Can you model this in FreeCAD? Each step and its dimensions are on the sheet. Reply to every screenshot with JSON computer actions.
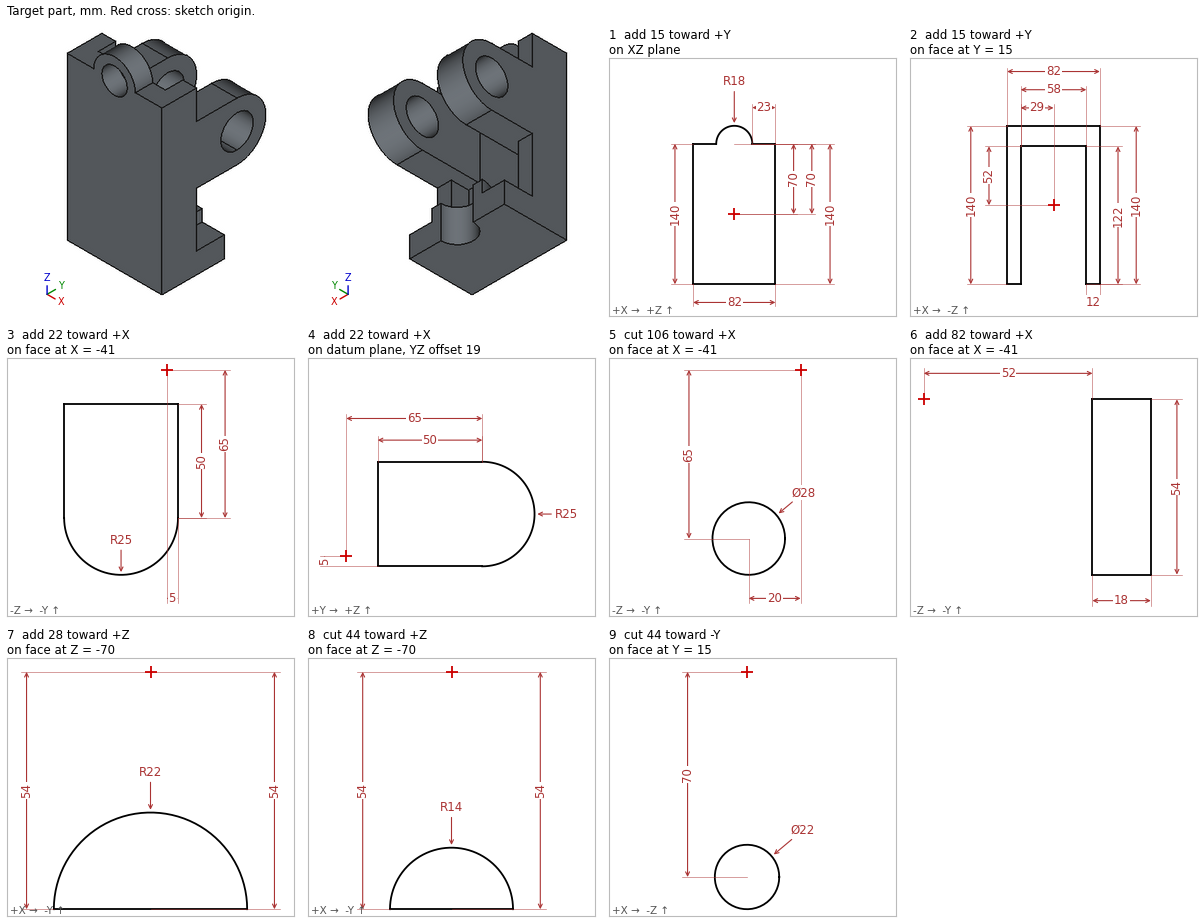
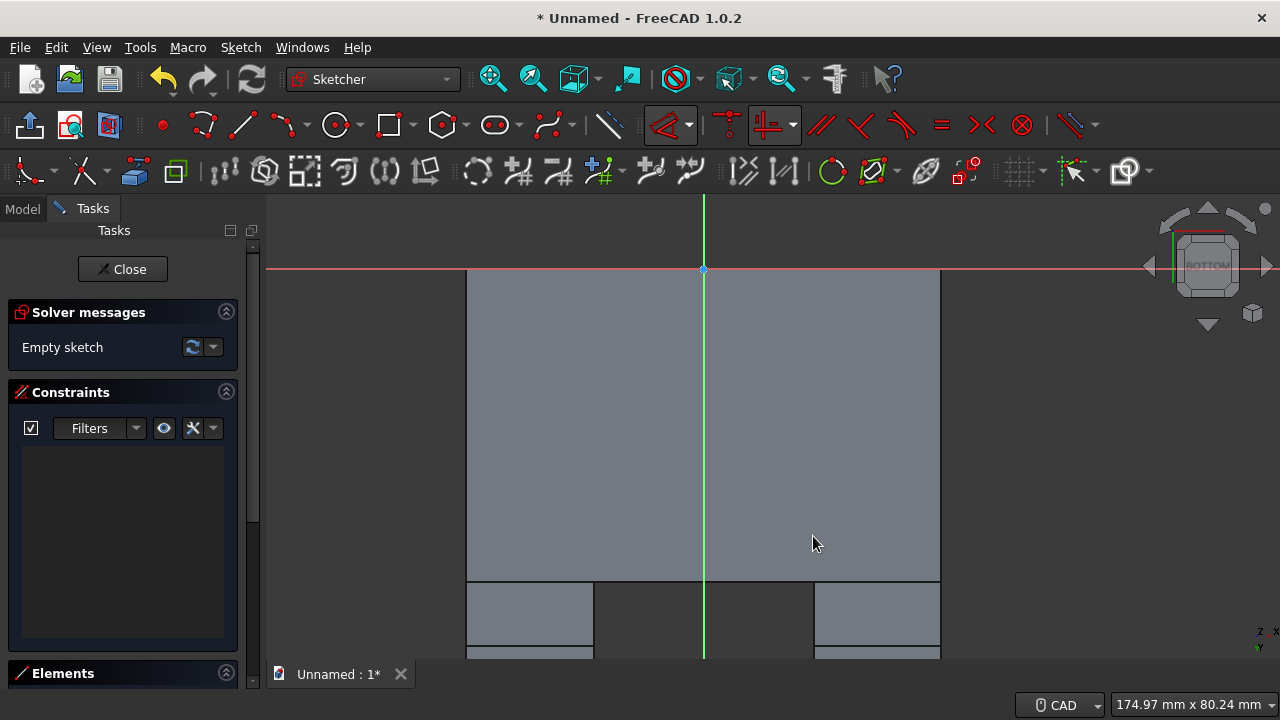
{"action": "key", "text": "g l"}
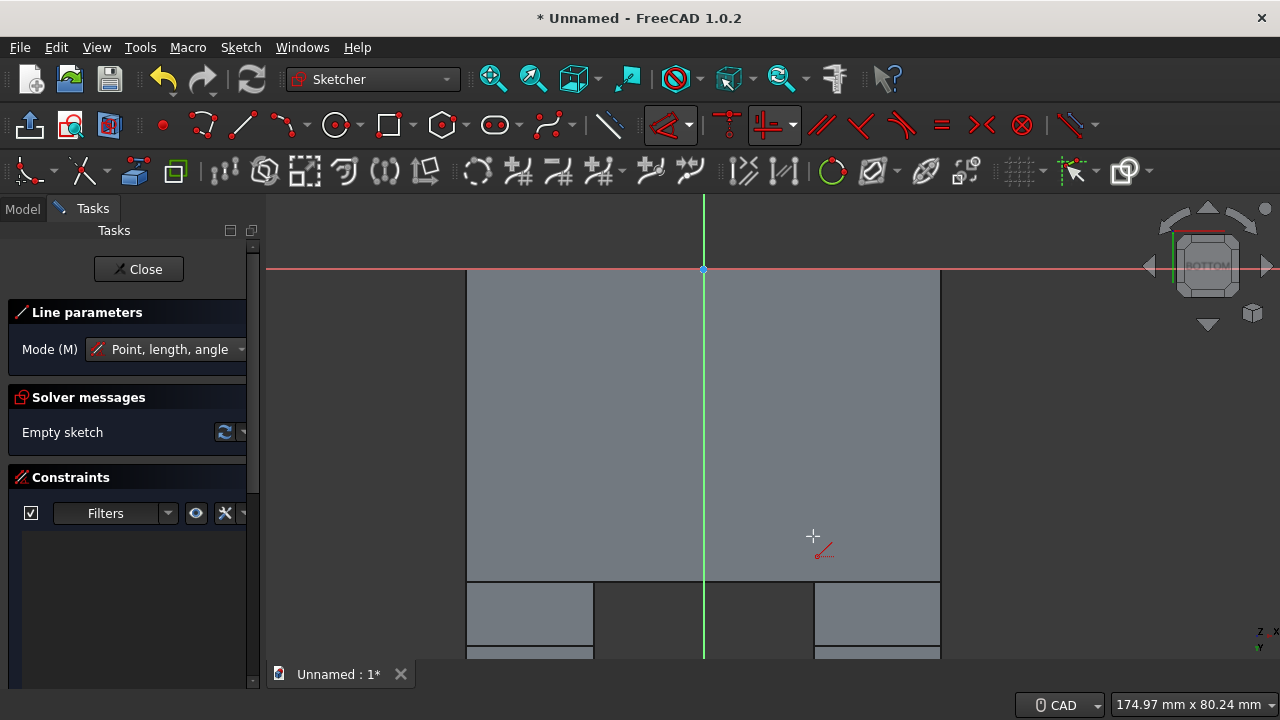
{"action": "left_click", "coordinate": [576, 582]}
{"action": "left_click", "coordinate": [831, 582]}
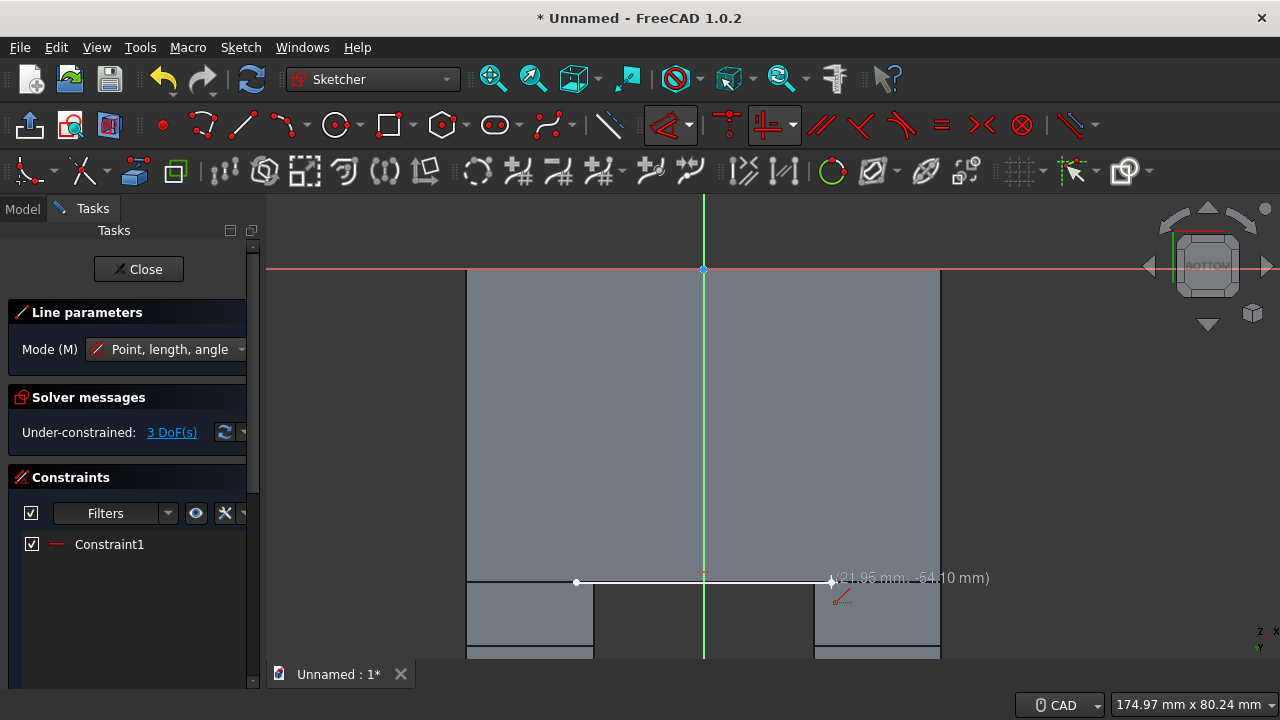
{"action": "left_click", "coordinate": [284, 126]}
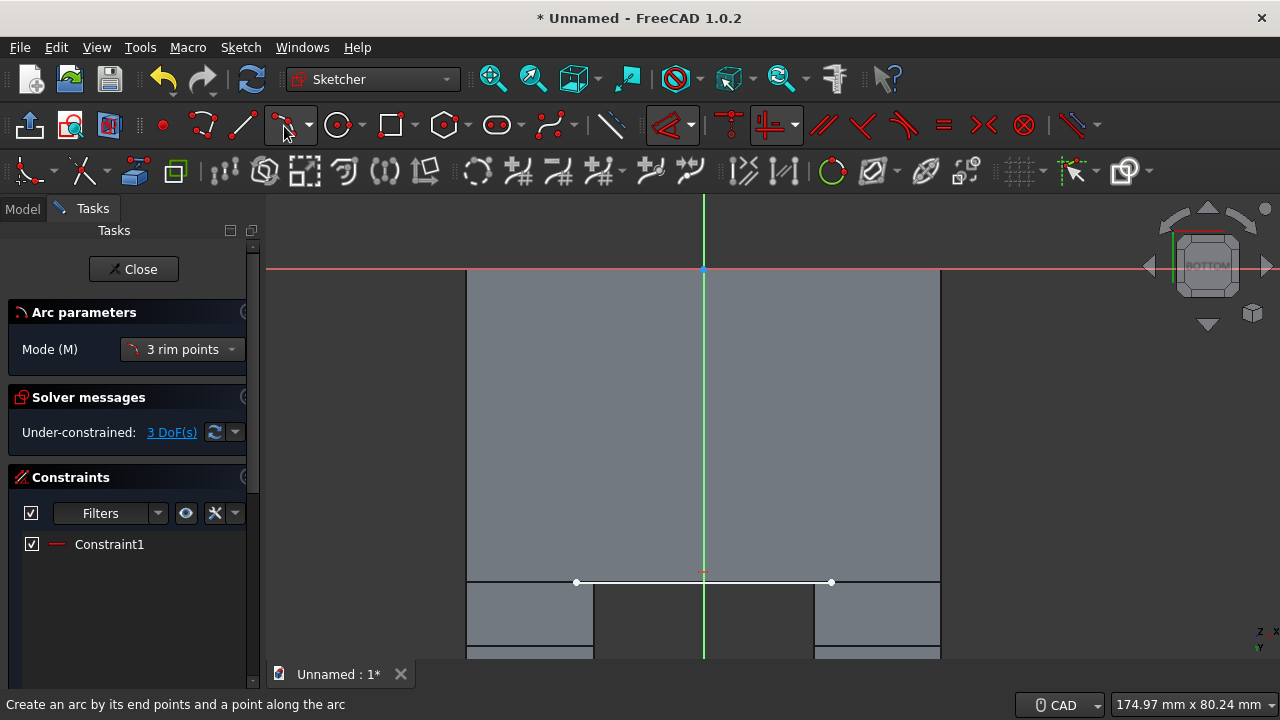
{"action": "left_click", "coordinate": [831, 583]}
{"action": "left_click", "coordinate": [576, 583]}
{"action": "left_click", "coordinate": [743, 461]}
{"action": "key", "text": "Escape"}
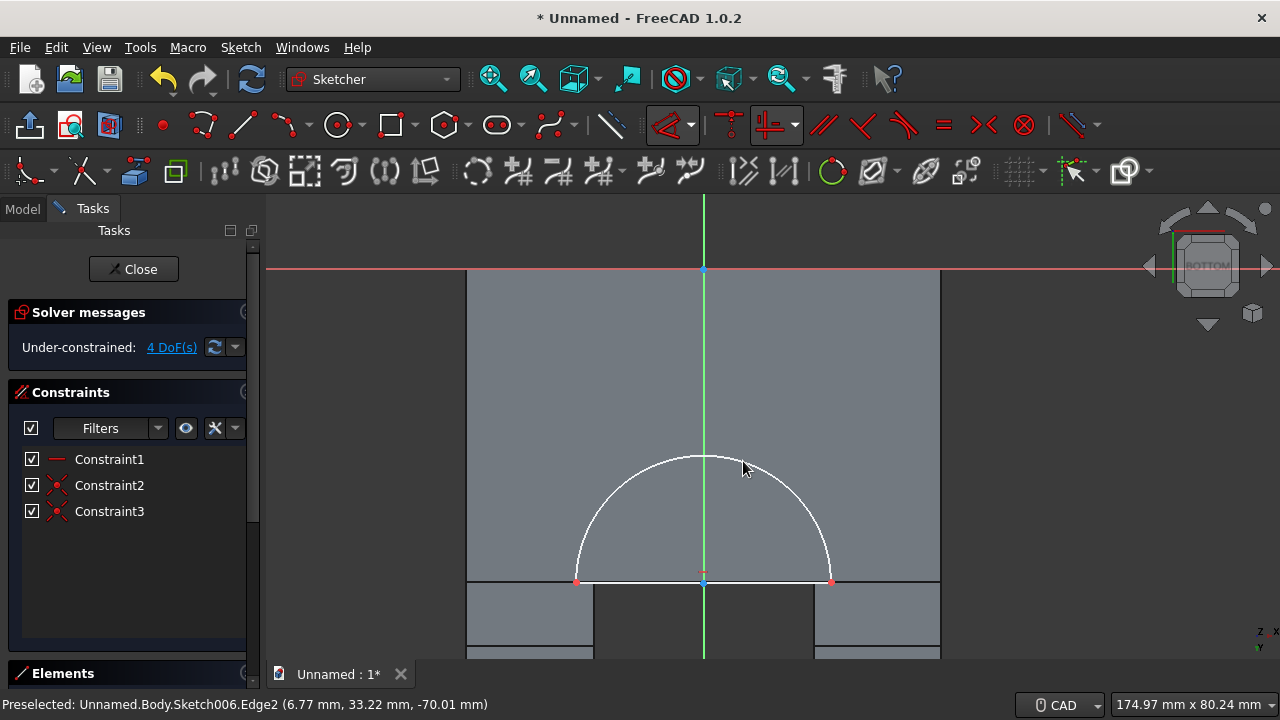
{"action": "left_click", "coordinate": [704, 583]}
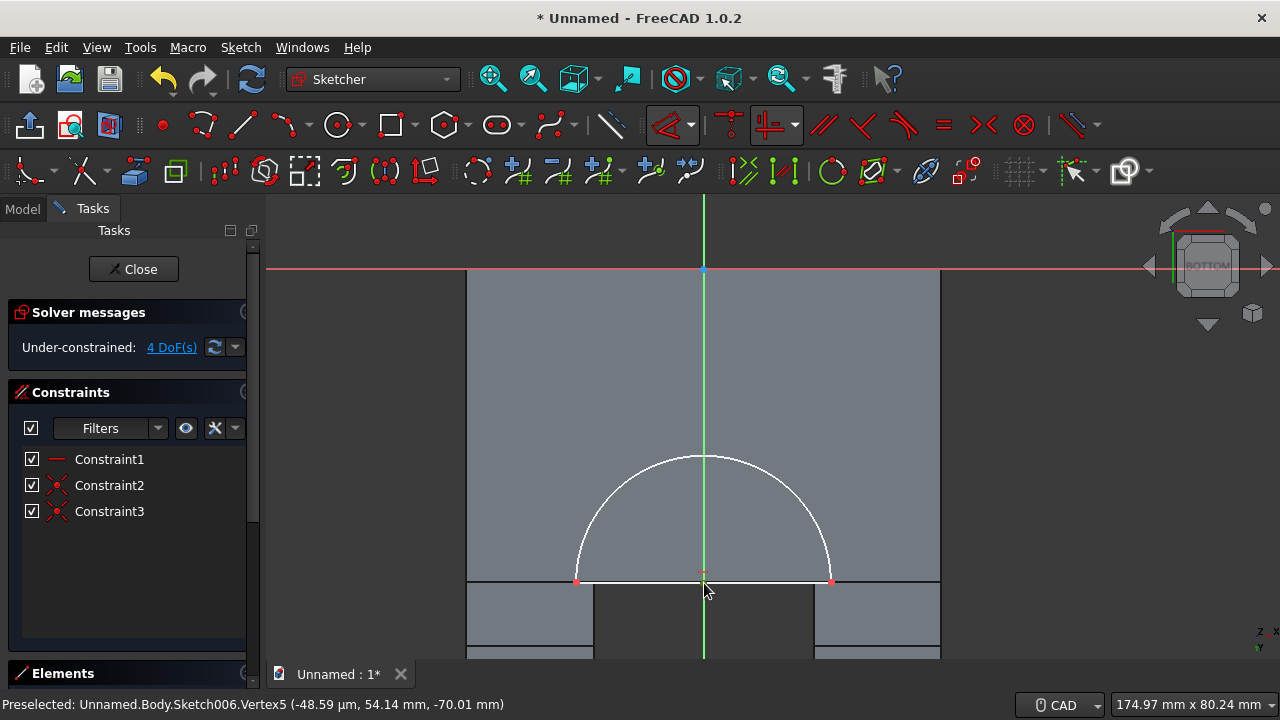
{"action": "left_click", "coordinate": [704, 543]}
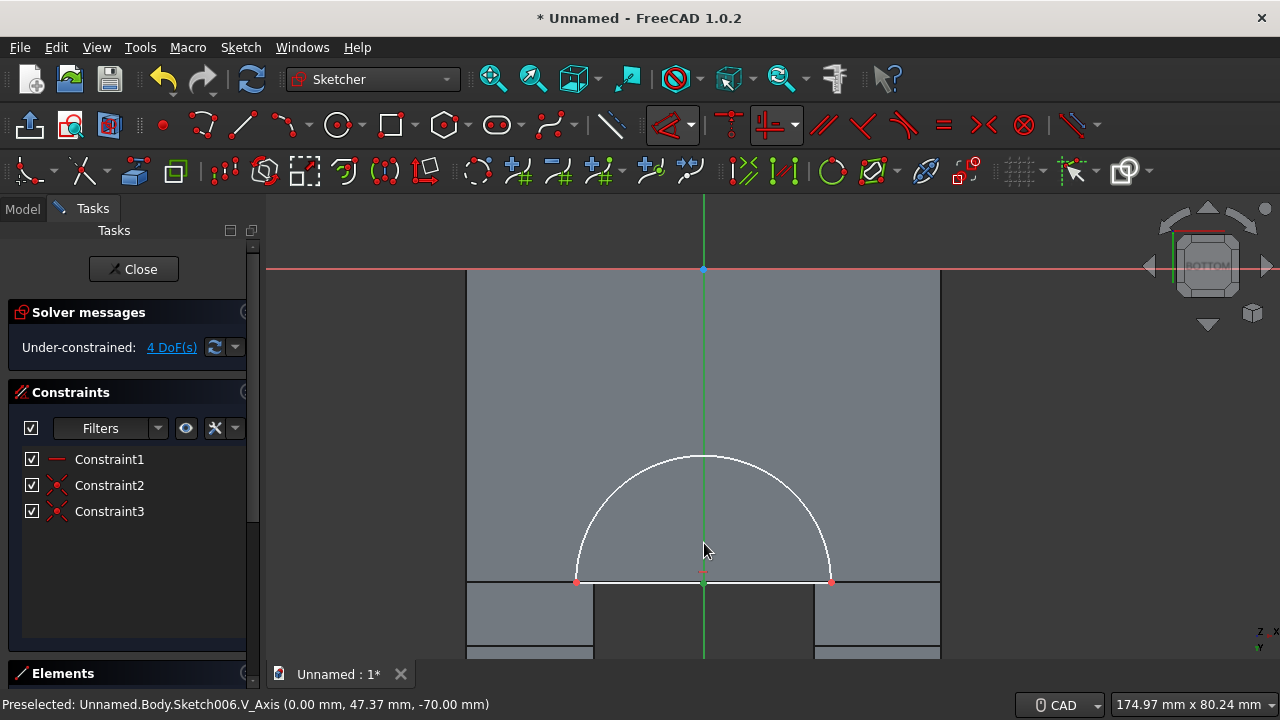
{"action": "left_click", "coordinate": [730, 126]}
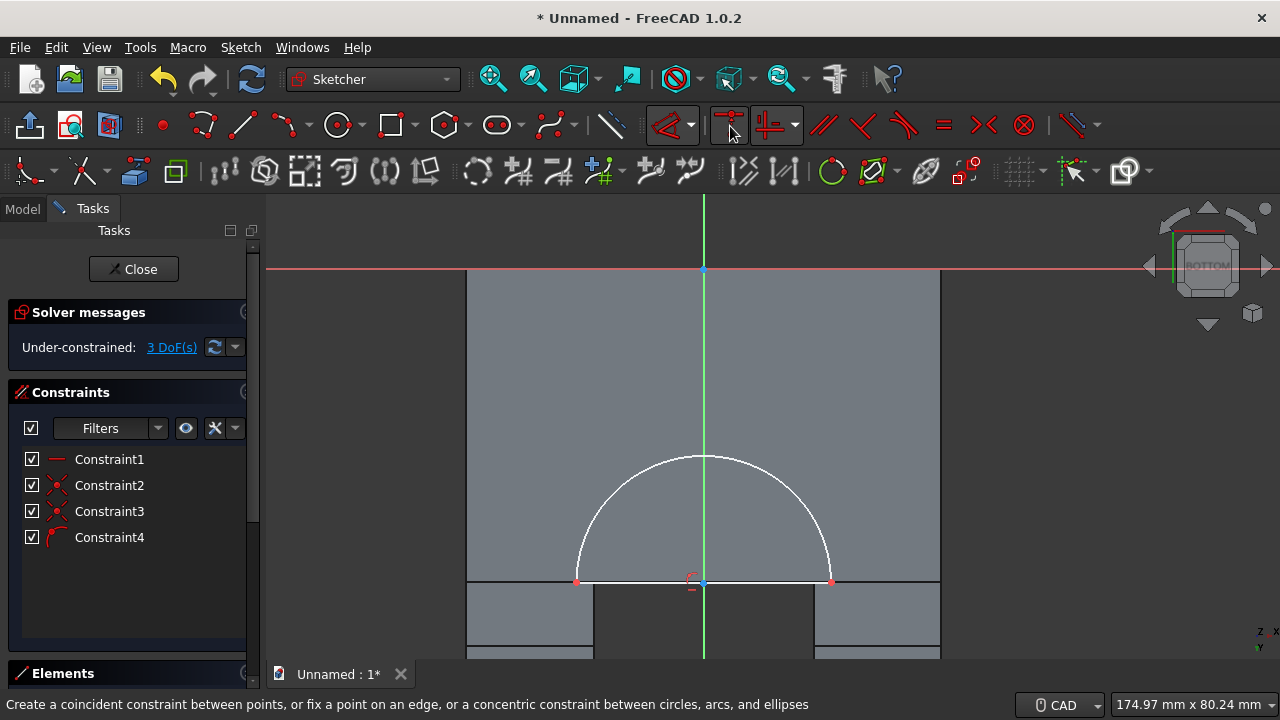
{"action": "left_click", "coordinate": [779, 480]}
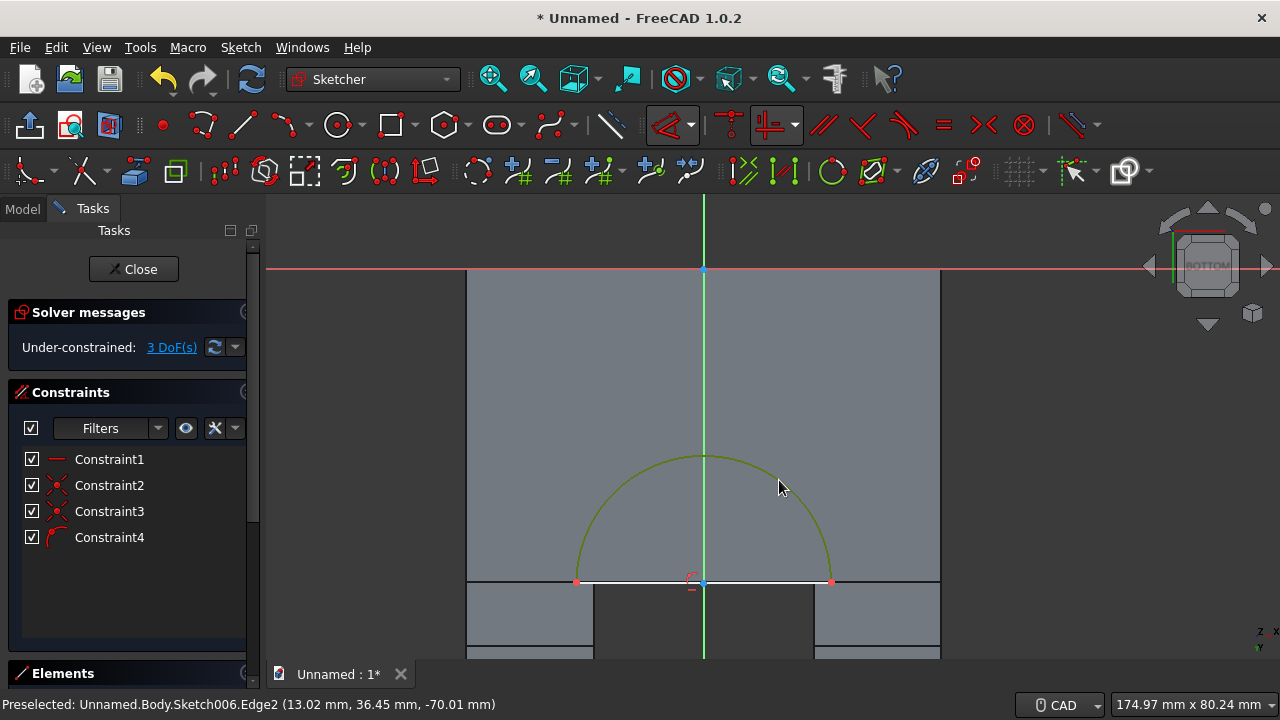
{"action": "key", "text": "k r"}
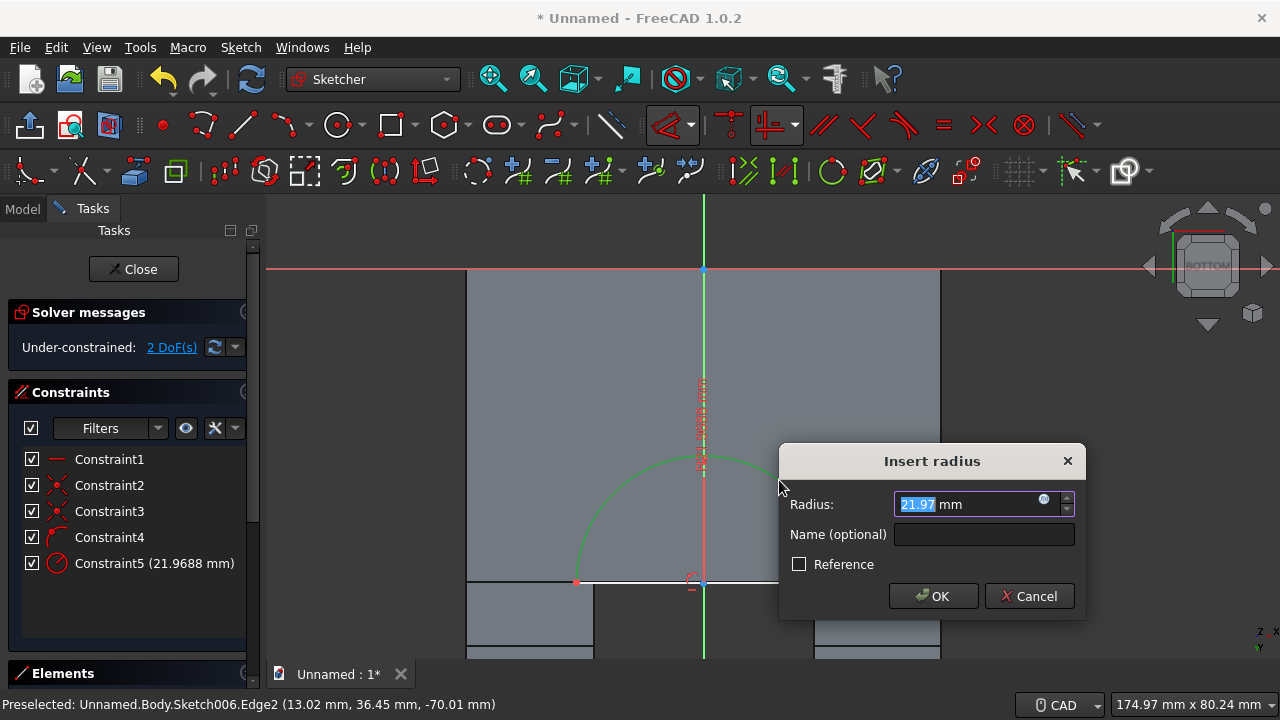
{"action": "type", "text": "22"}
{"action": "key", "text": "Return"}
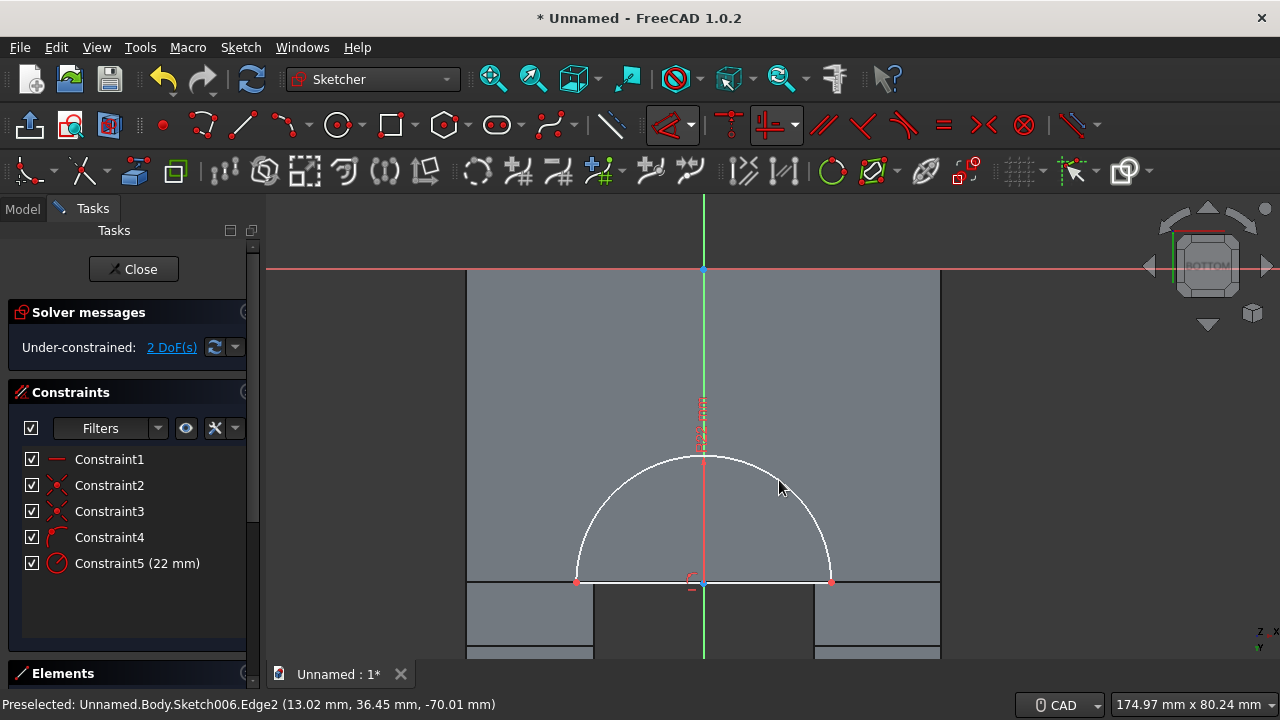
{"action": "left_click", "coordinate": [576, 583]}